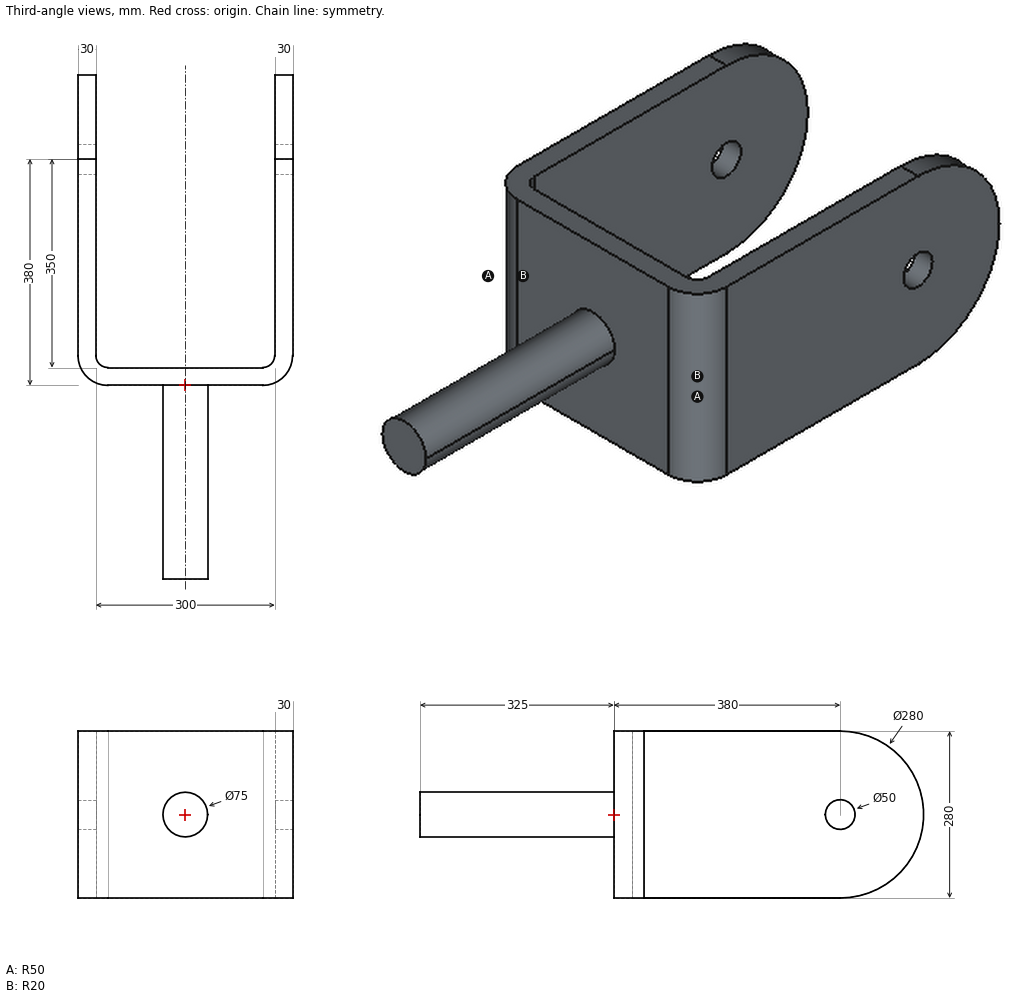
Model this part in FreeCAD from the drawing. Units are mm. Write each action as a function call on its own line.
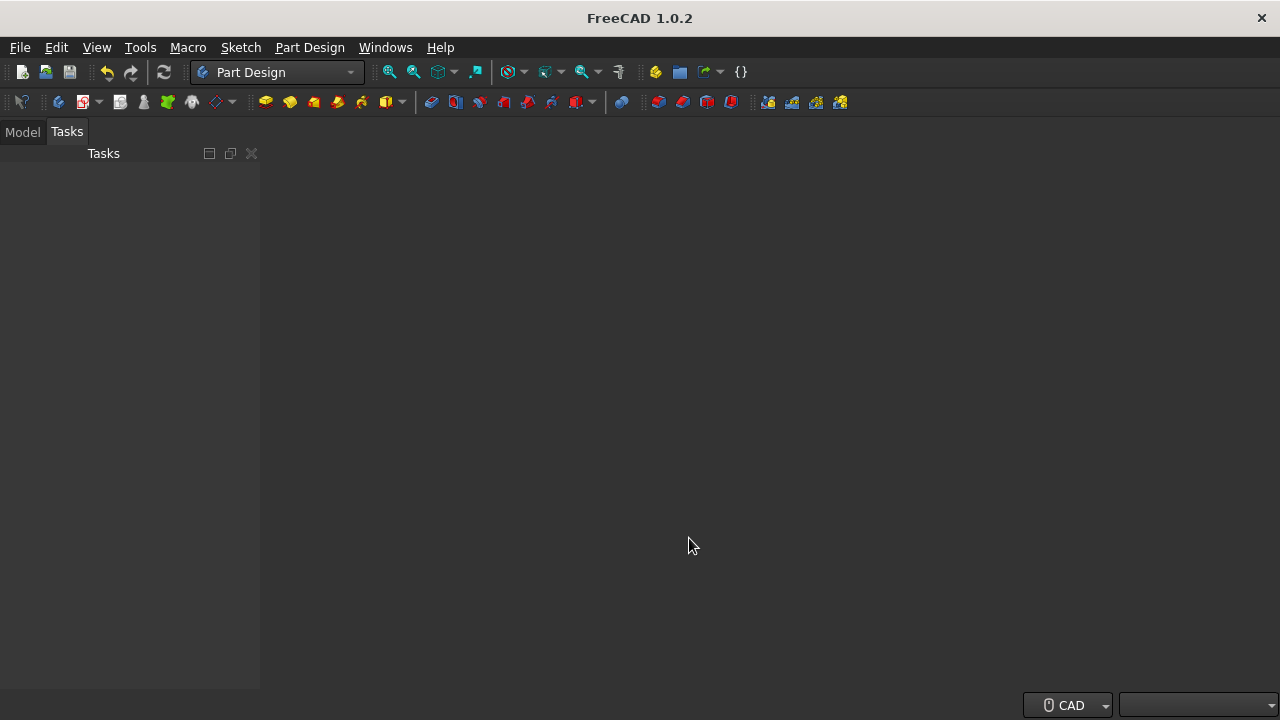
click(22, 72)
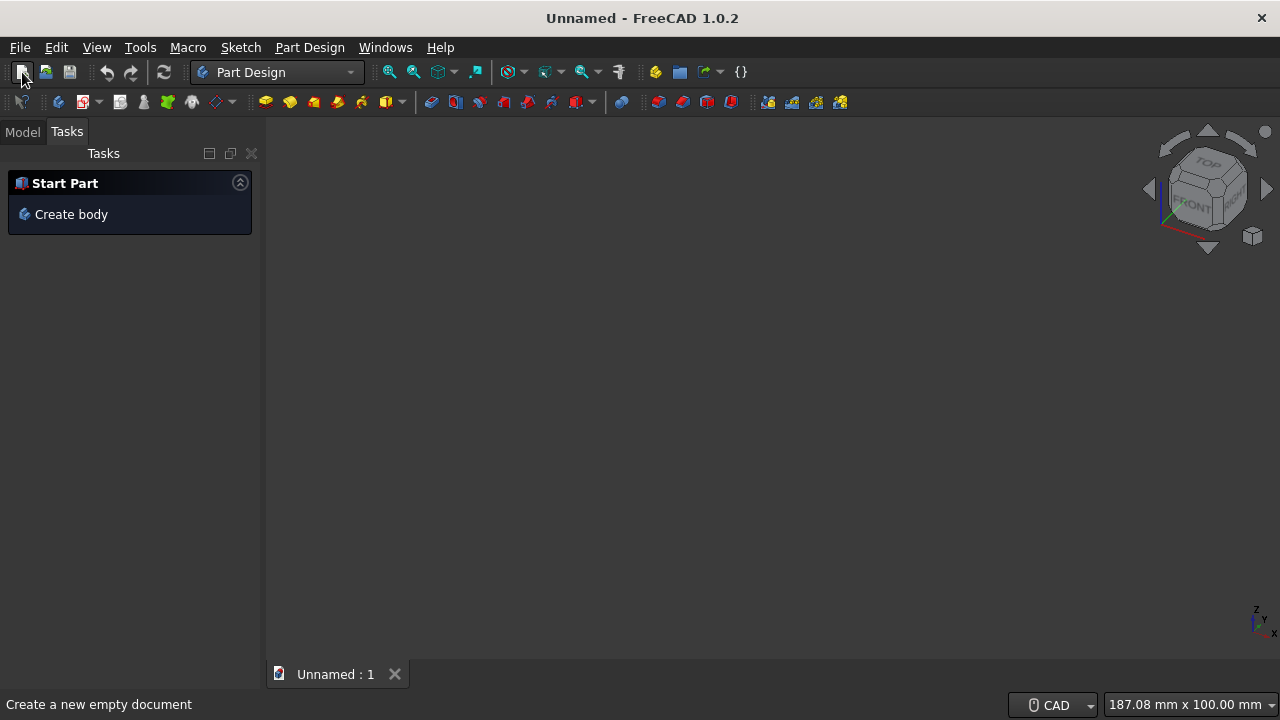
click(84, 102)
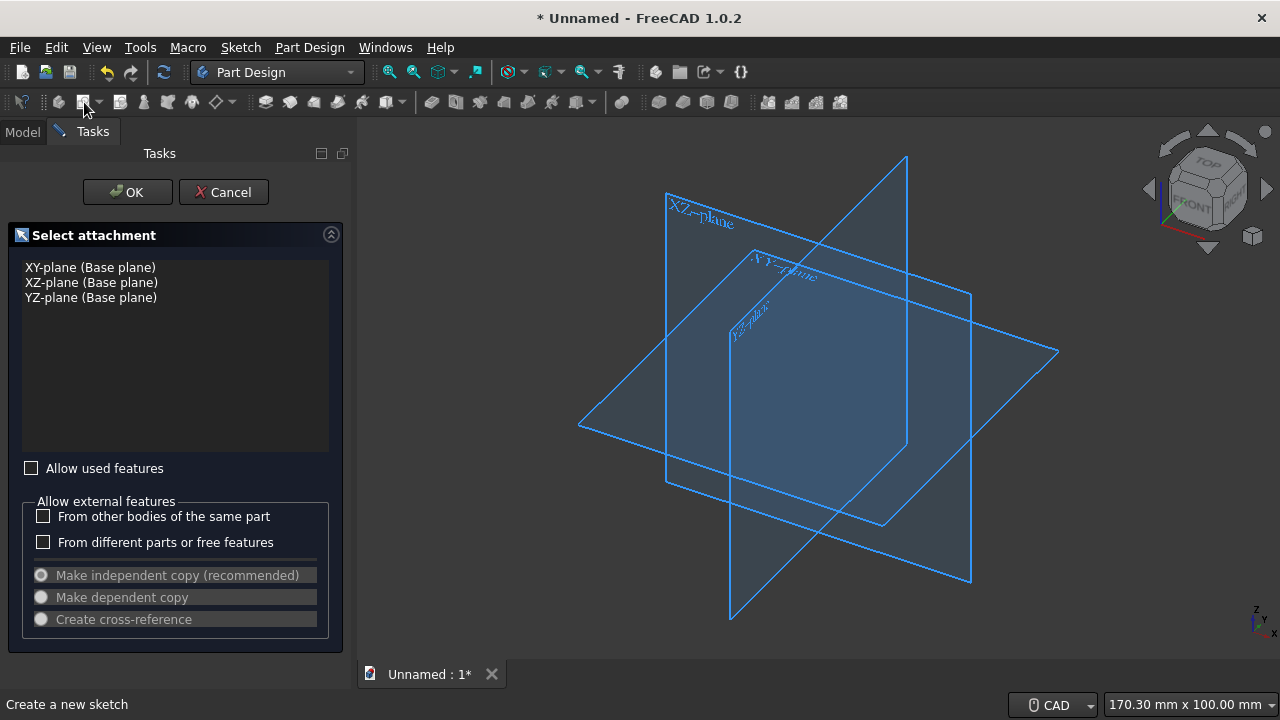
click(82, 268)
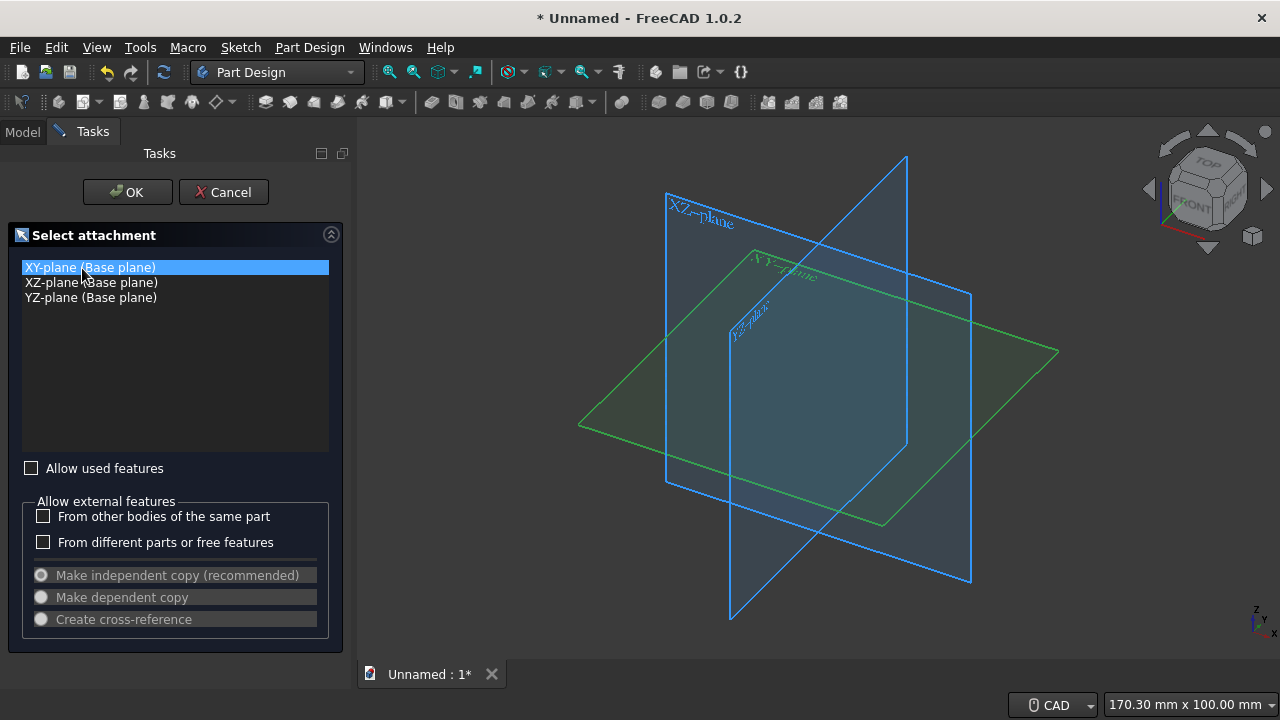
click(128, 192)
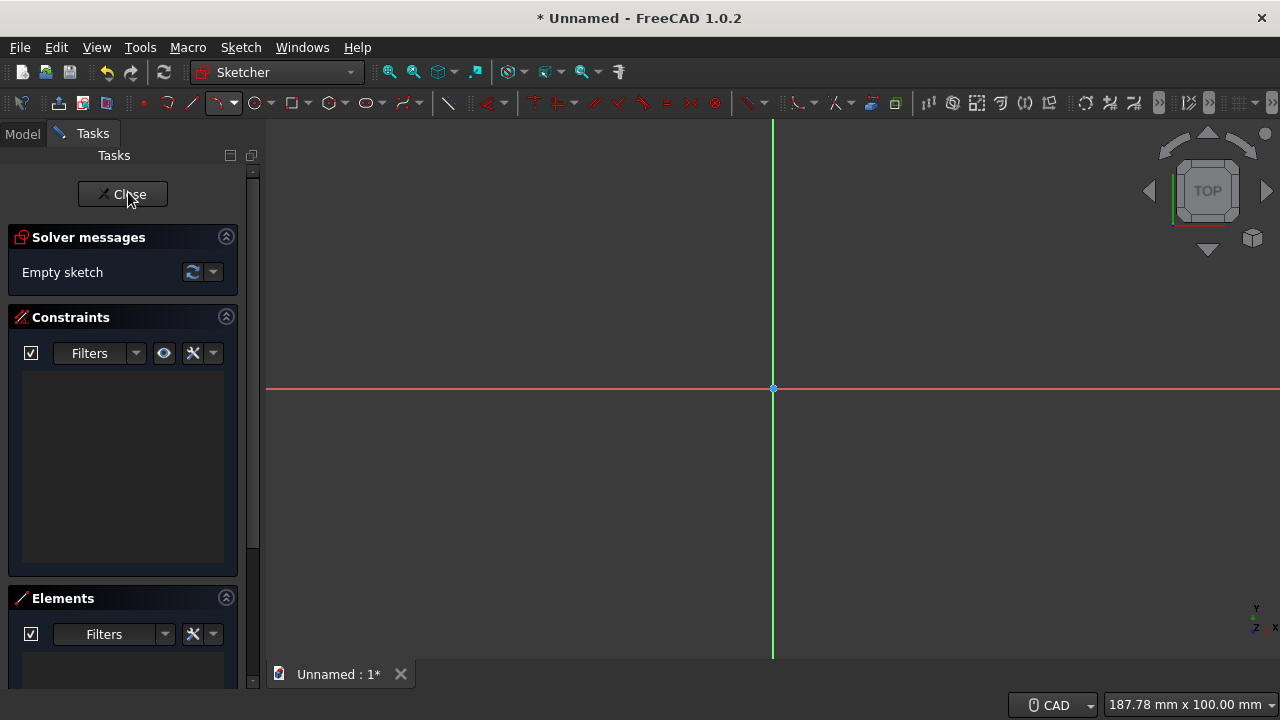
scroll(691, 592, down, 9)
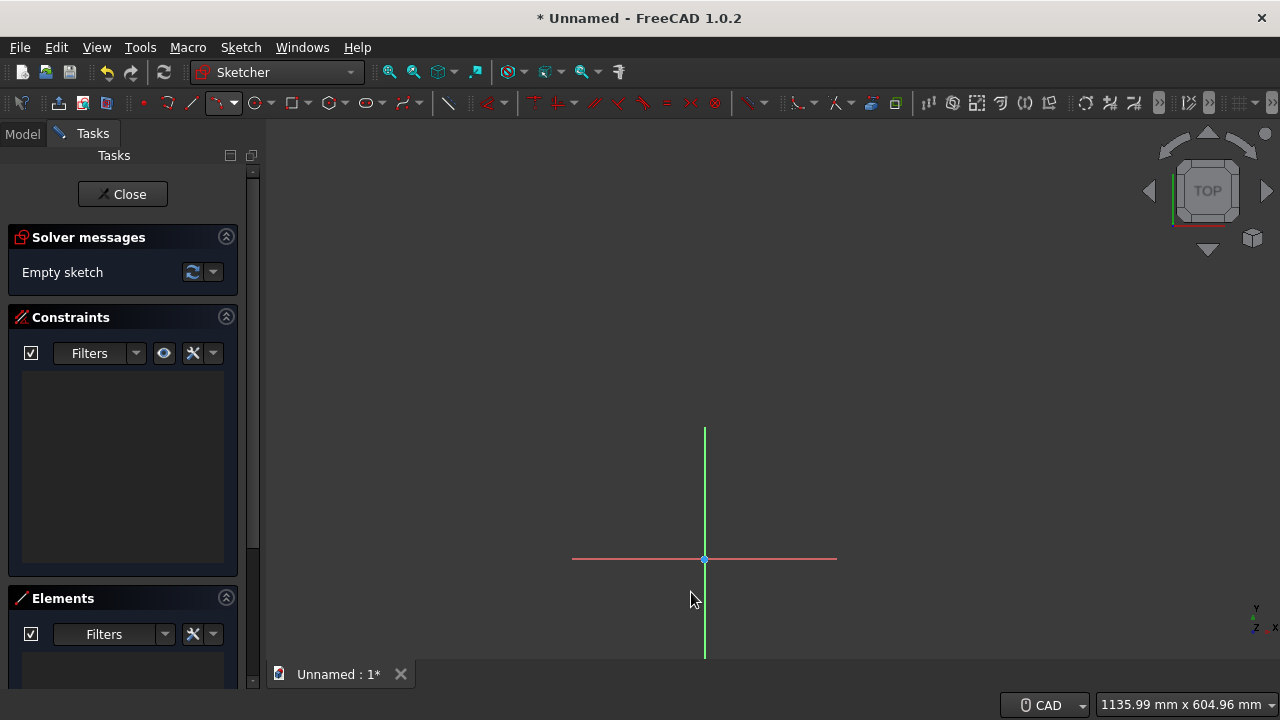
click(168, 104)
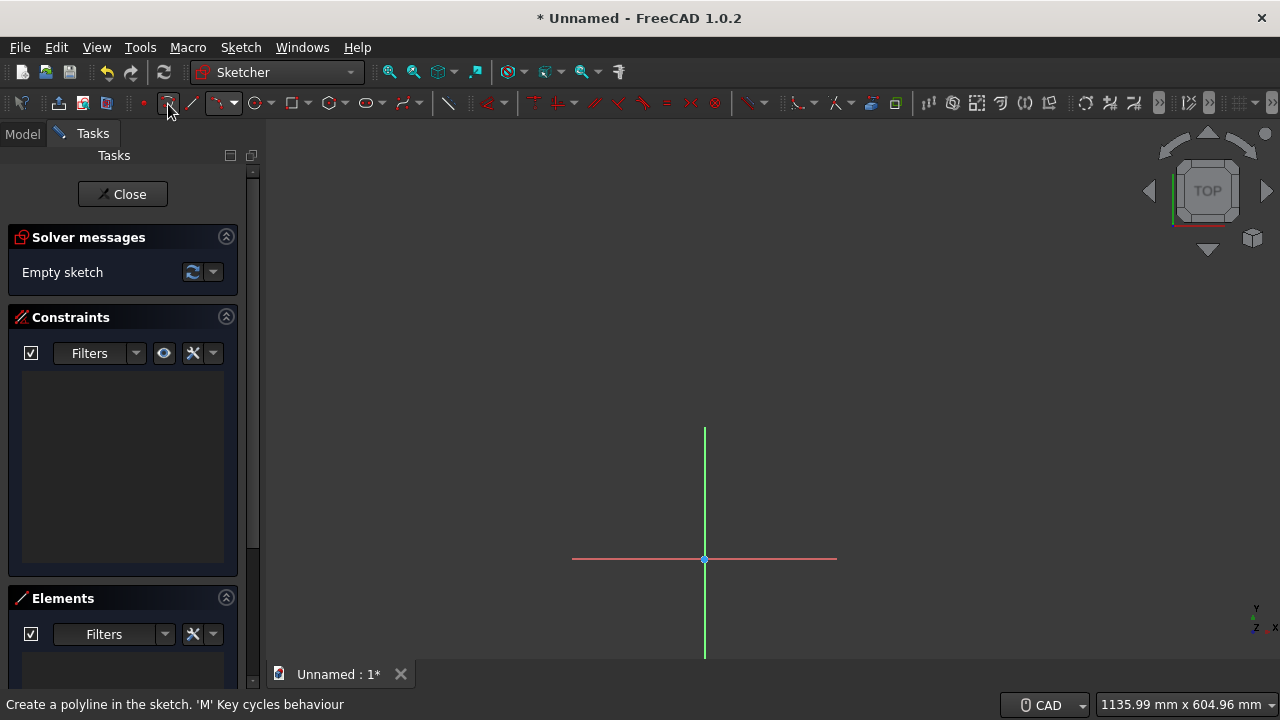
click(839, 532)
click(571, 532)
click(571, 220)
click(544, 220)
click(544, 559)
click(866, 550)
click(866, 220)
click(839, 220)
click(839, 533)
key(Escape)
key(Escape)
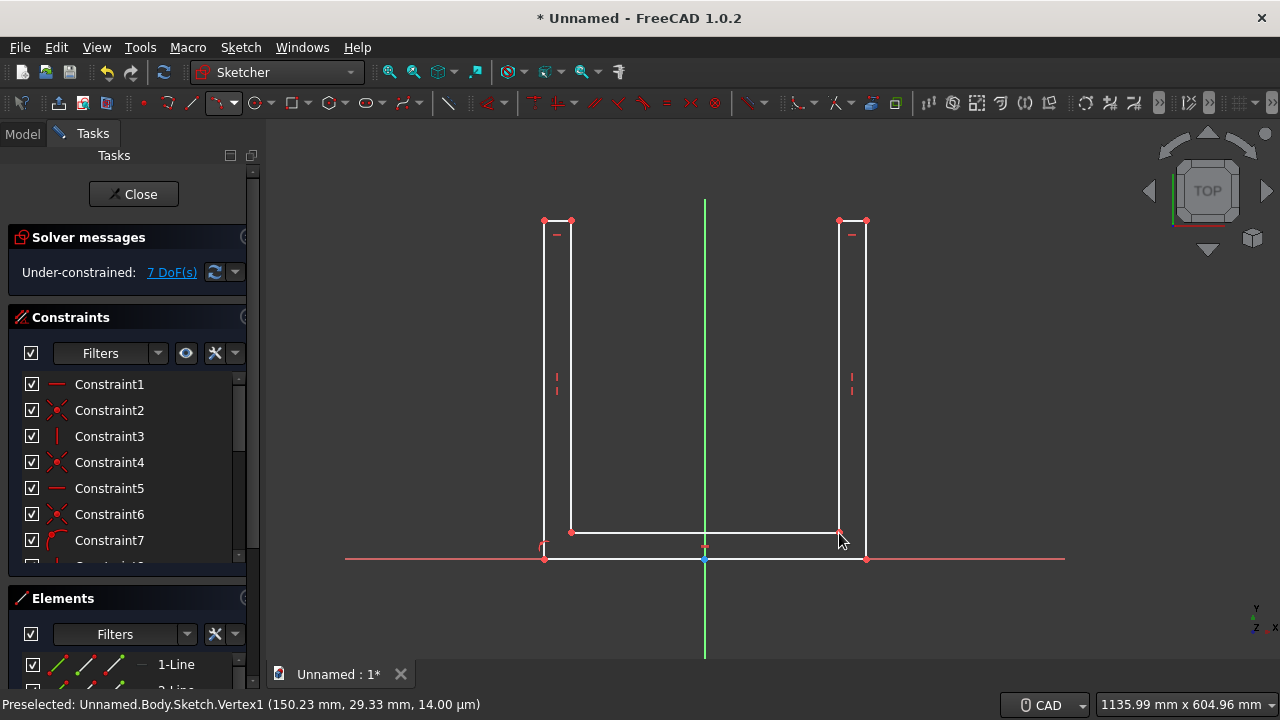
click(544, 221)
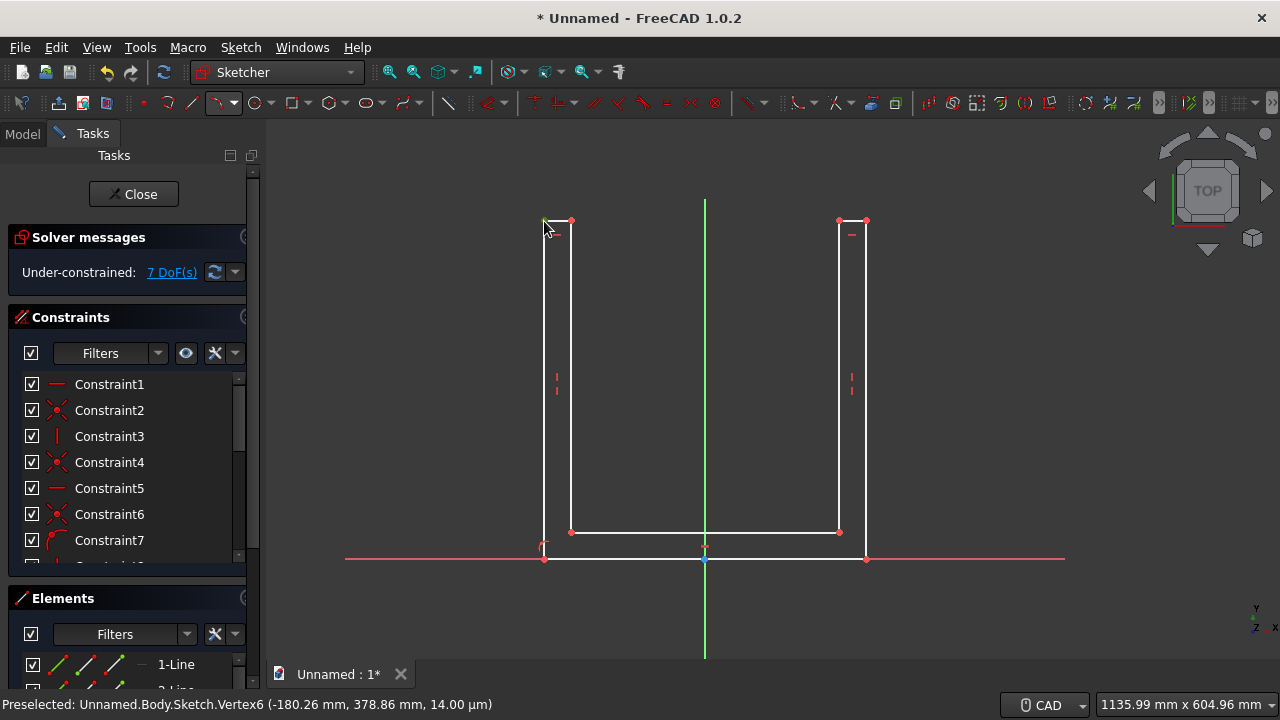
click(866, 221)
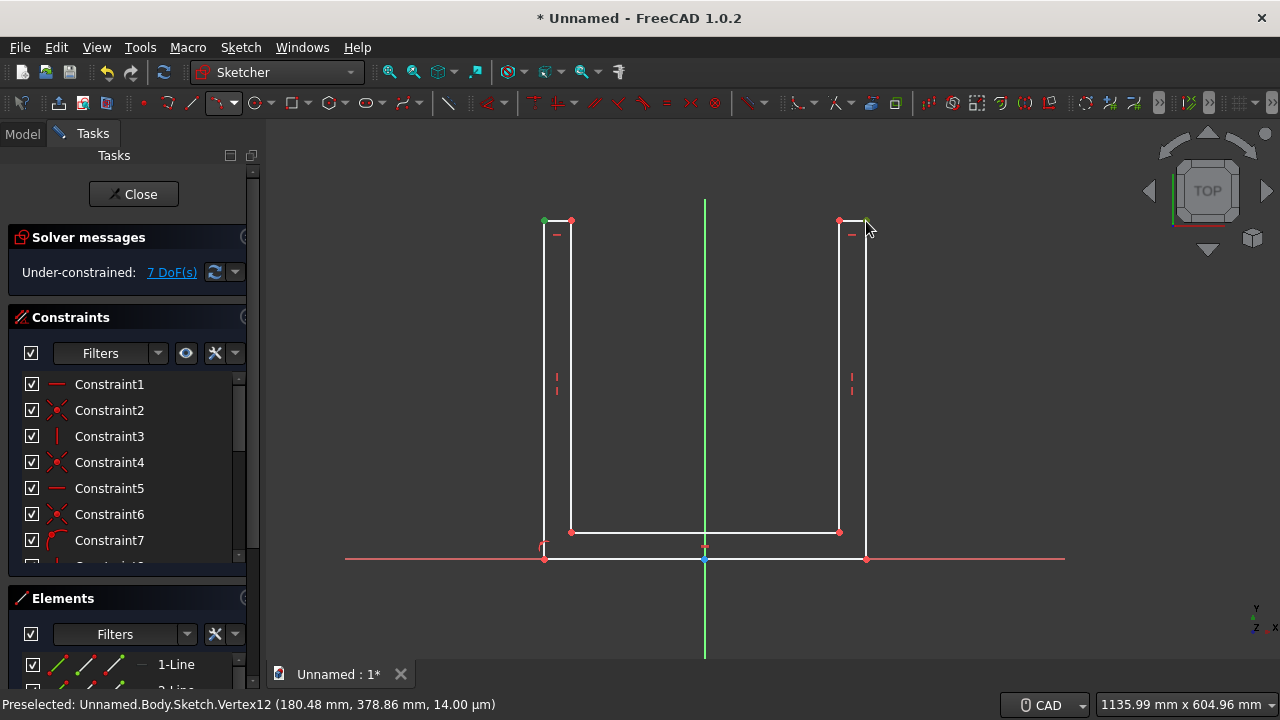
click(705, 596)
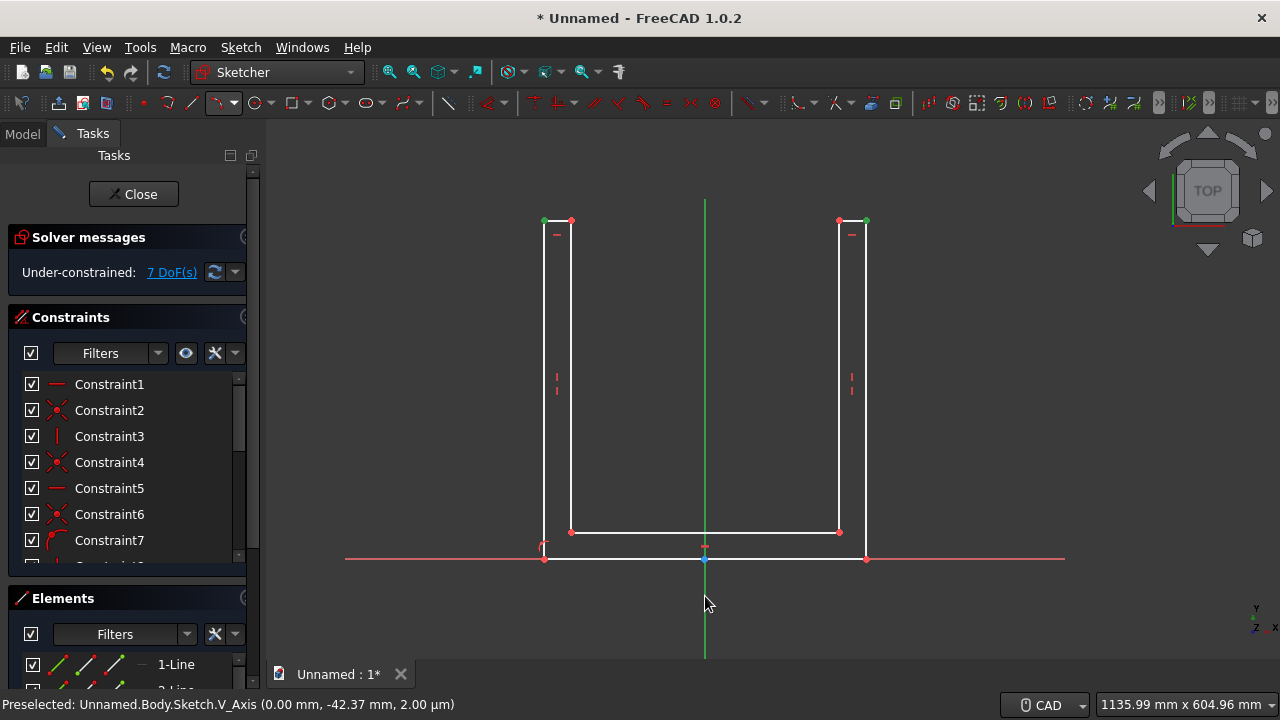
click(692, 104)